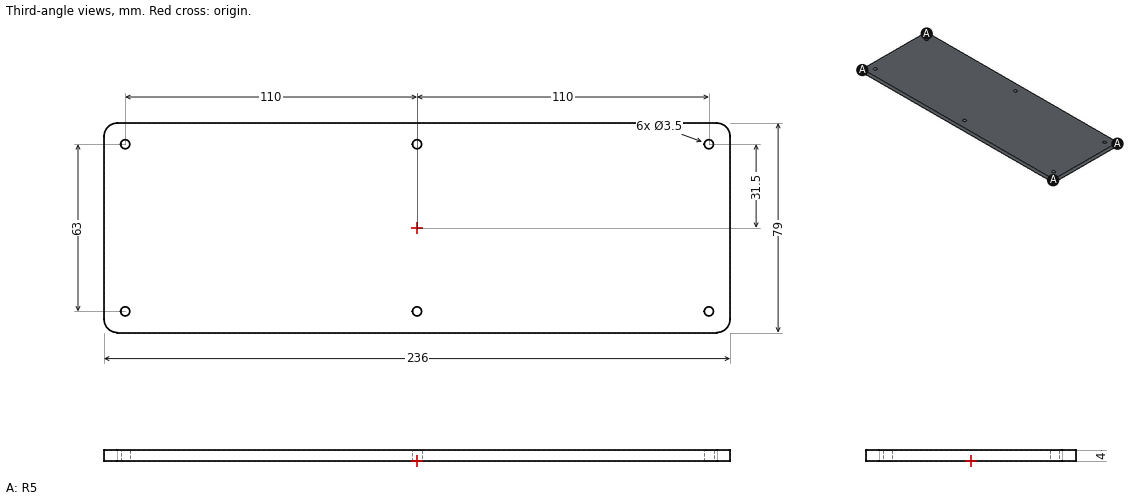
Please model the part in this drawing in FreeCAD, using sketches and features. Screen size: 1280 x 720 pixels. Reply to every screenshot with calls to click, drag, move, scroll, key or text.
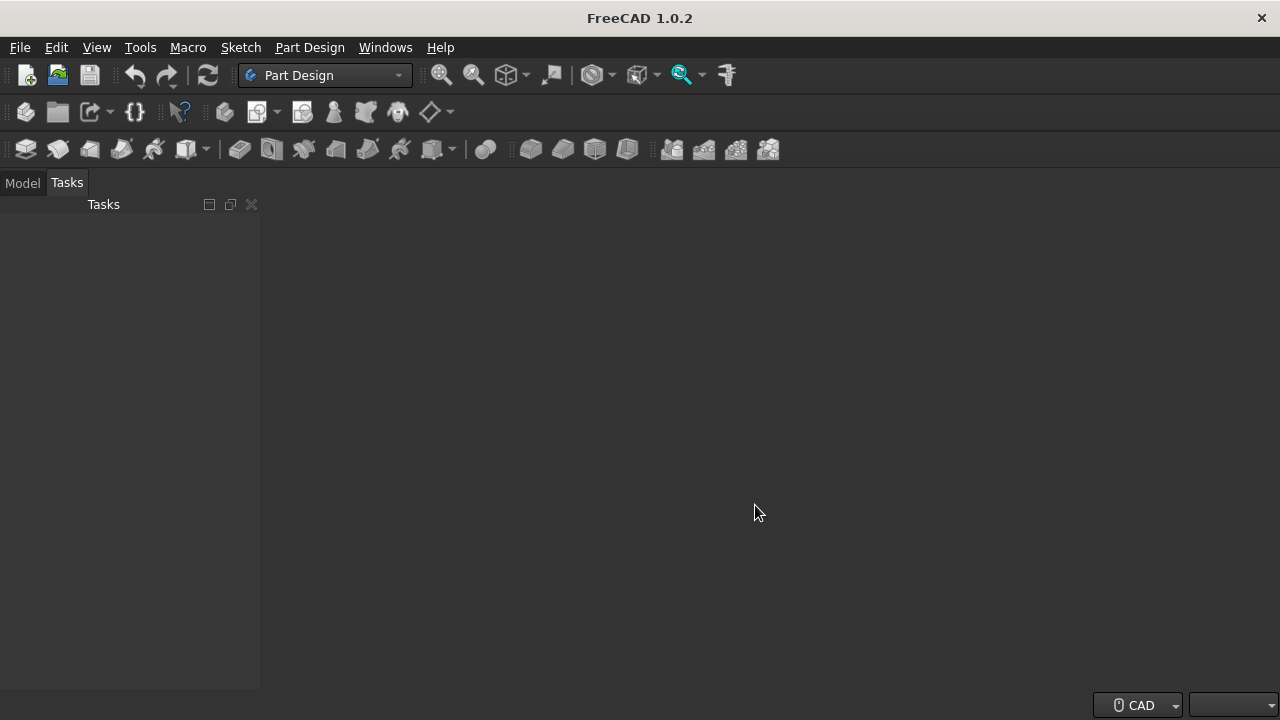
click(26, 76)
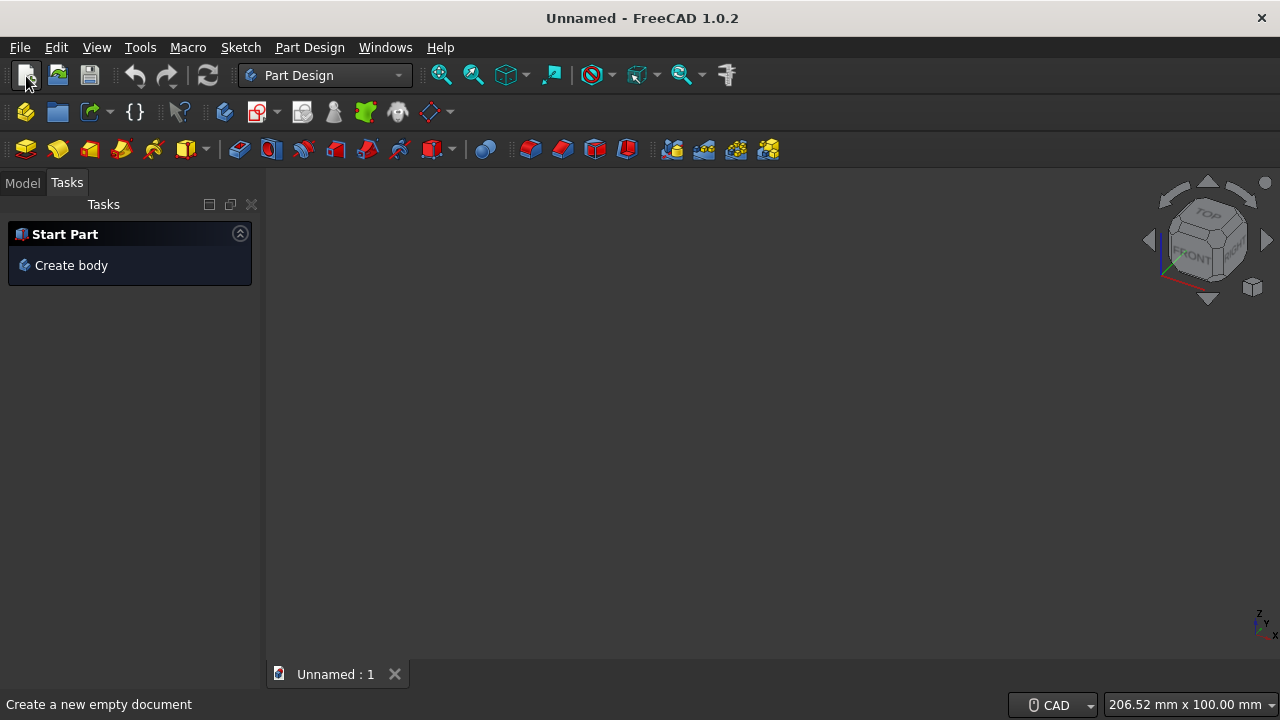
click(258, 112)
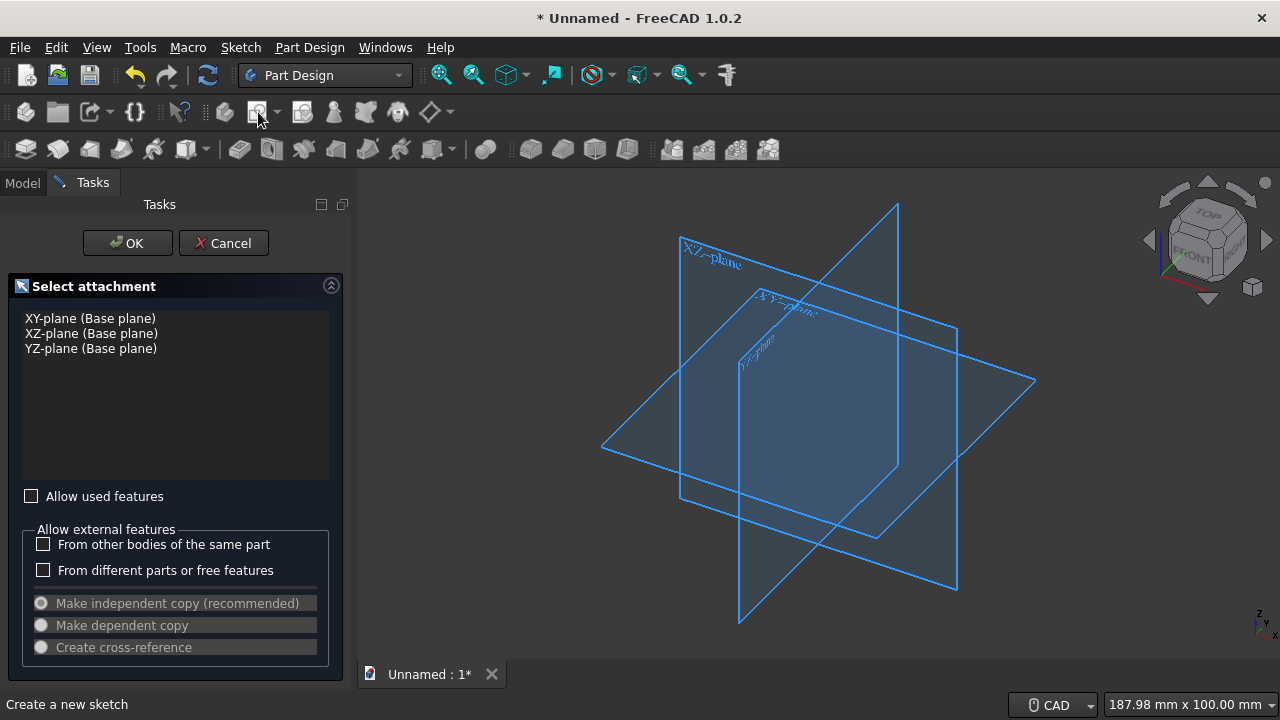
click(82, 318)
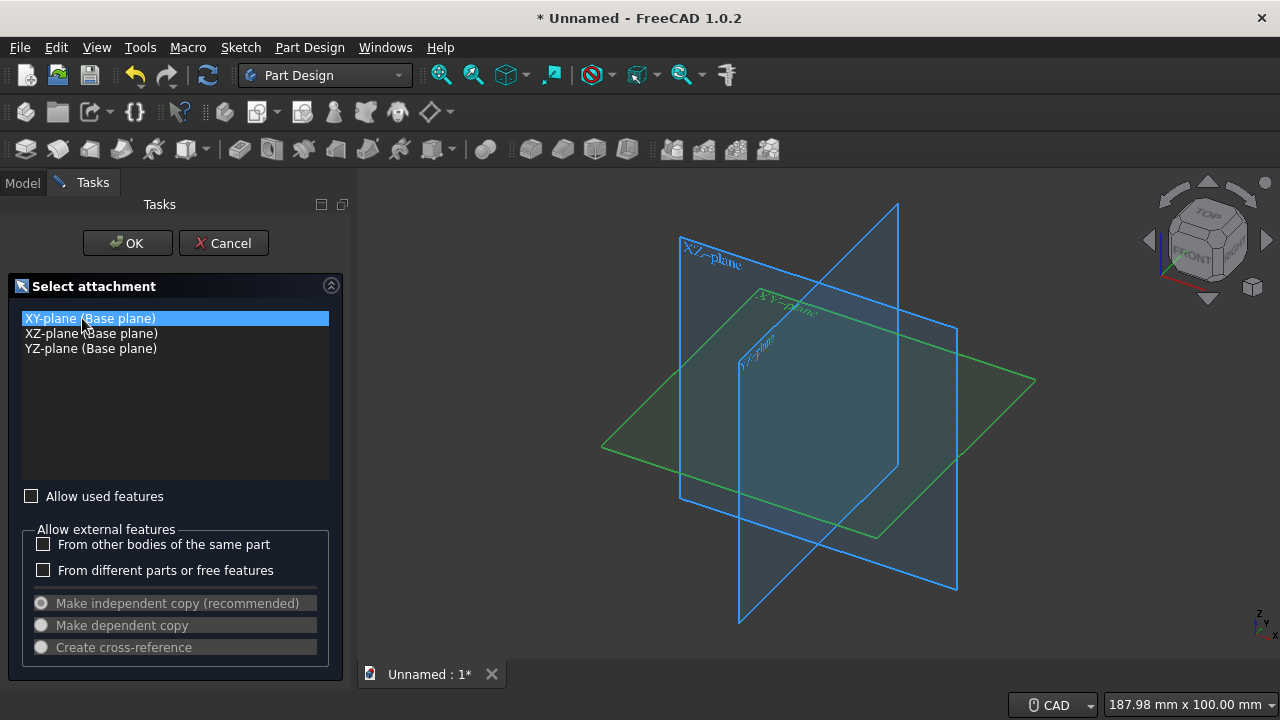
click(128, 243)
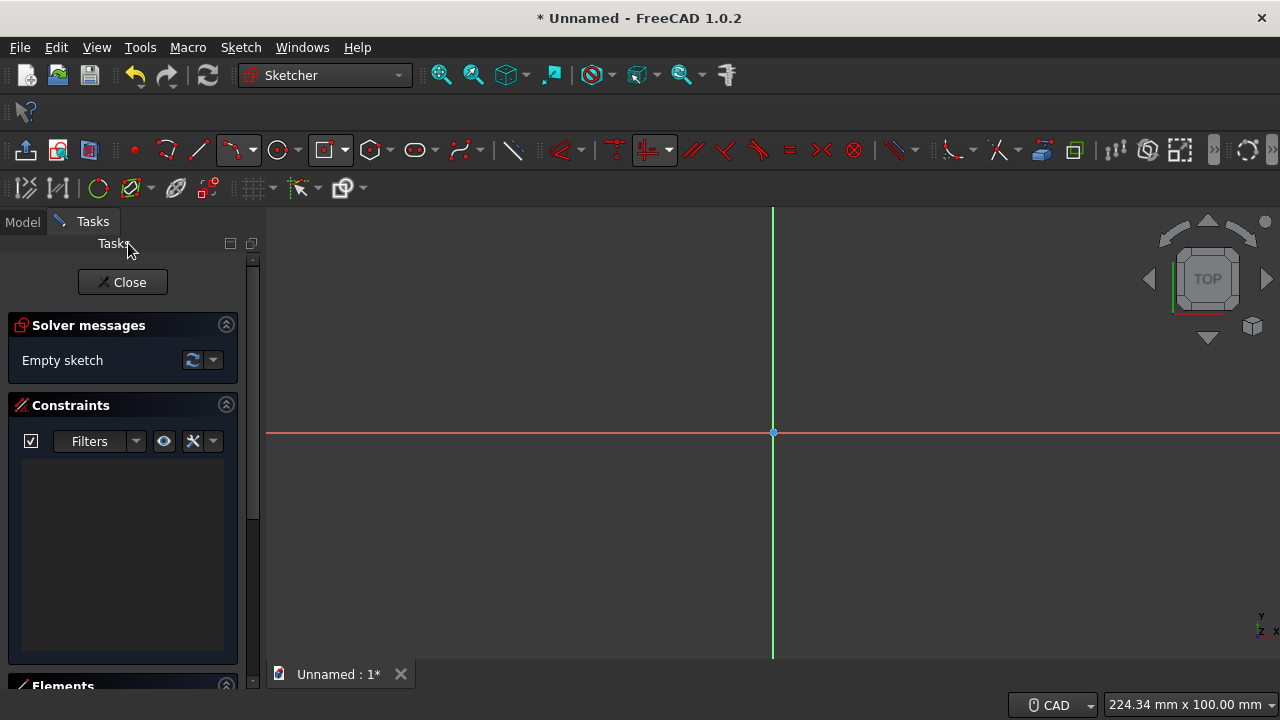
scroll(621, 433, down, 3)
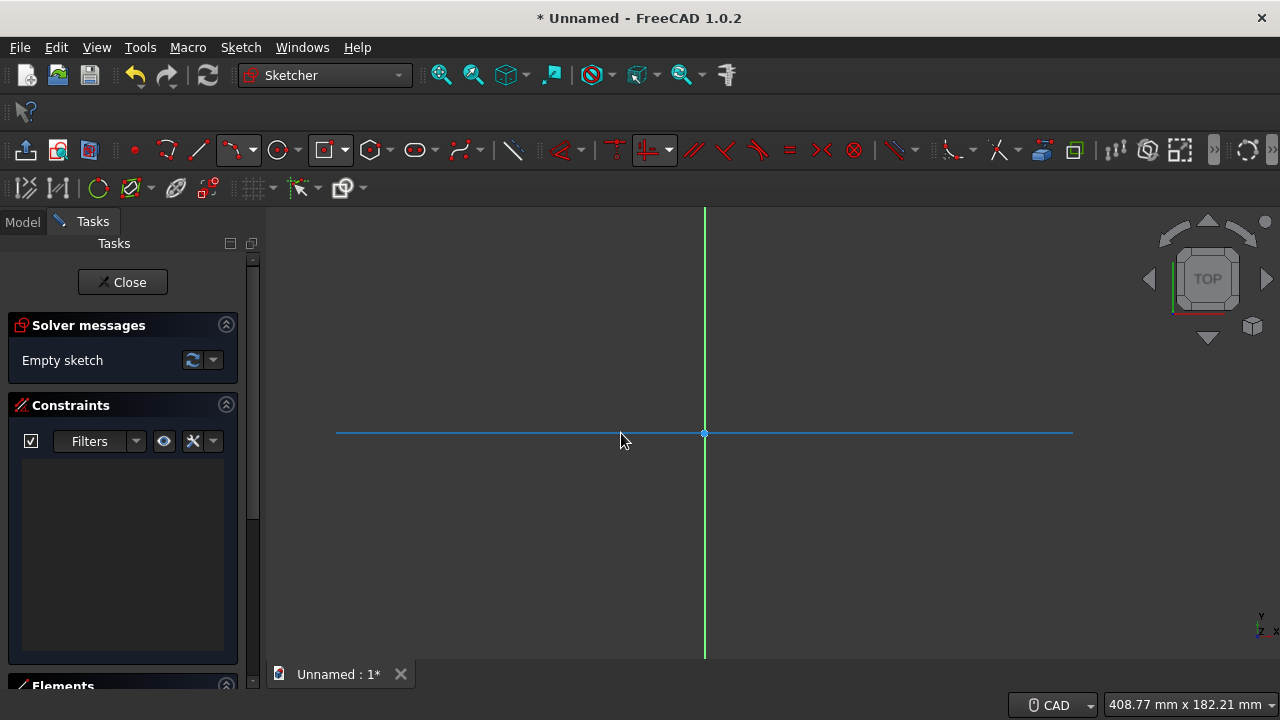
click(324, 150)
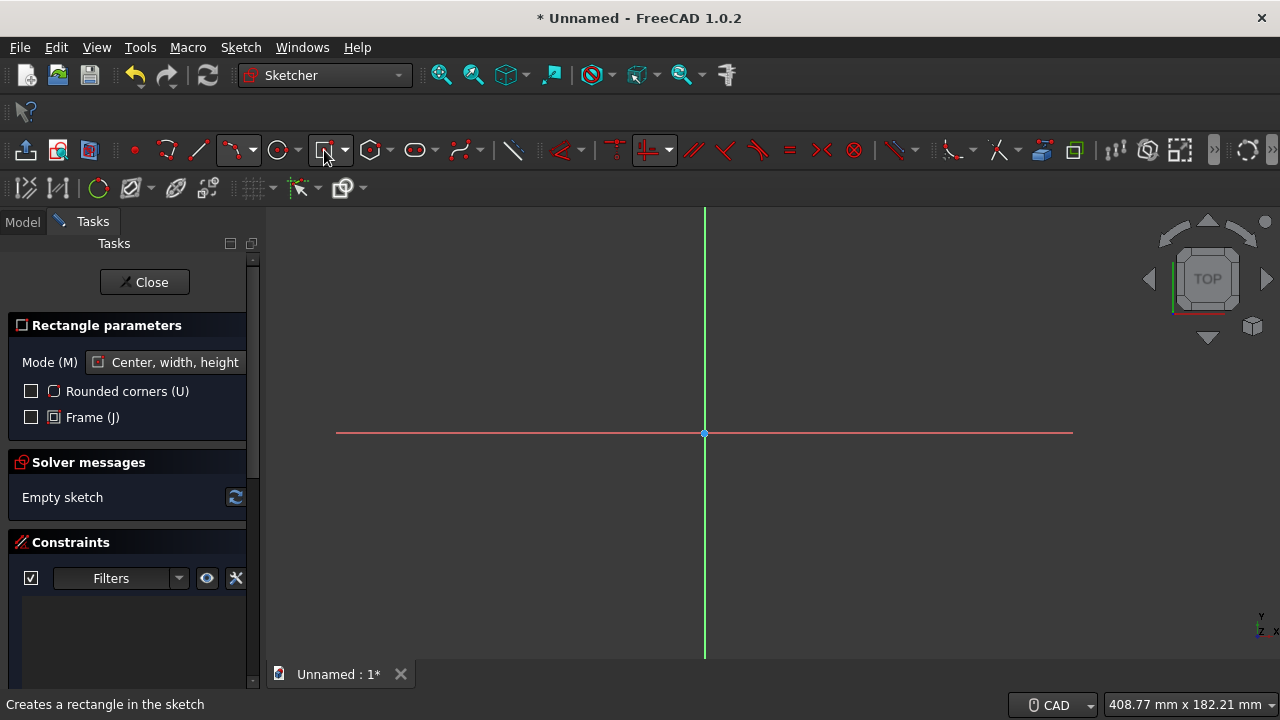
click(705, 433)
move(997, 335)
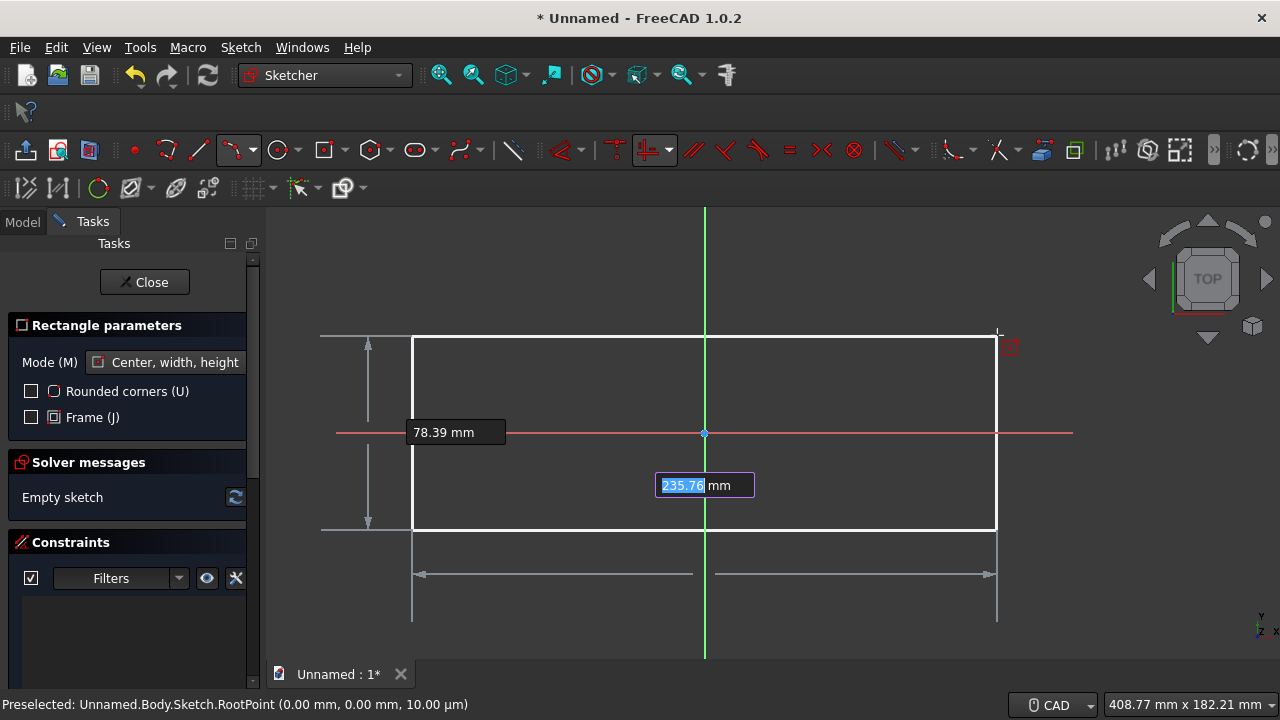
text(236)
key(Tab)
text(79)
key(Return)
key(Escape)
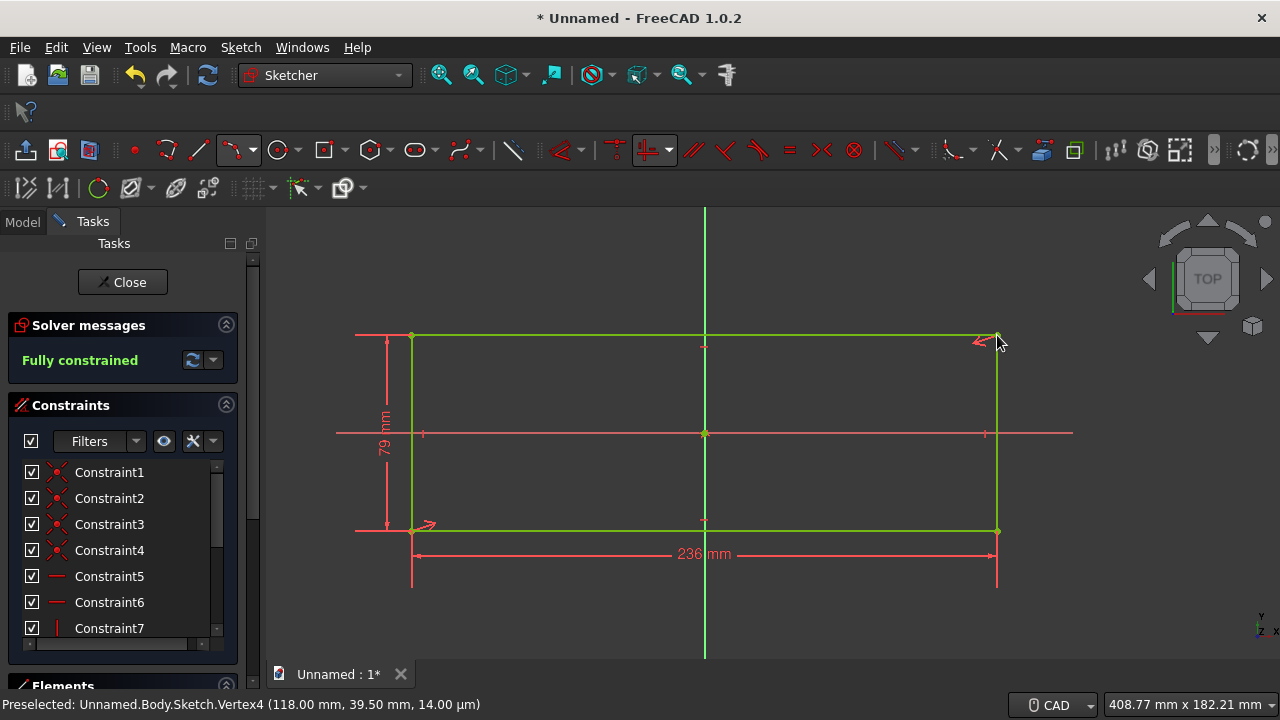
click(123, 282)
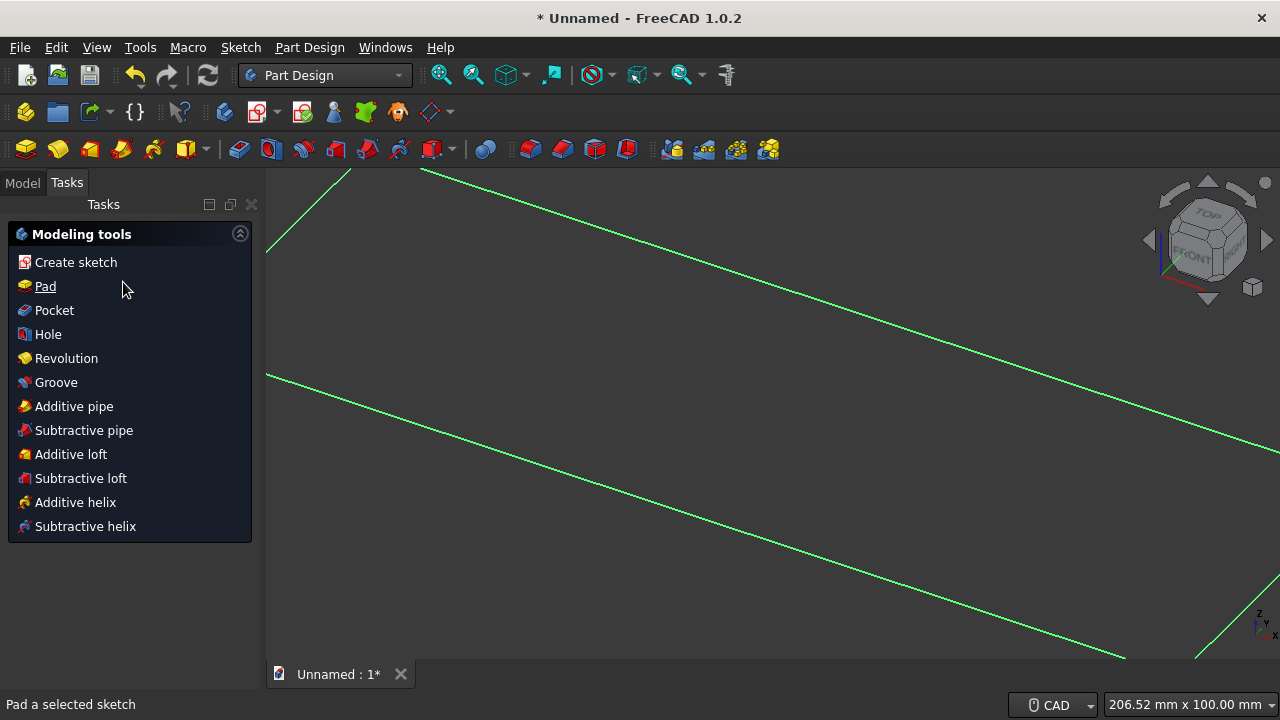
click(26, 150)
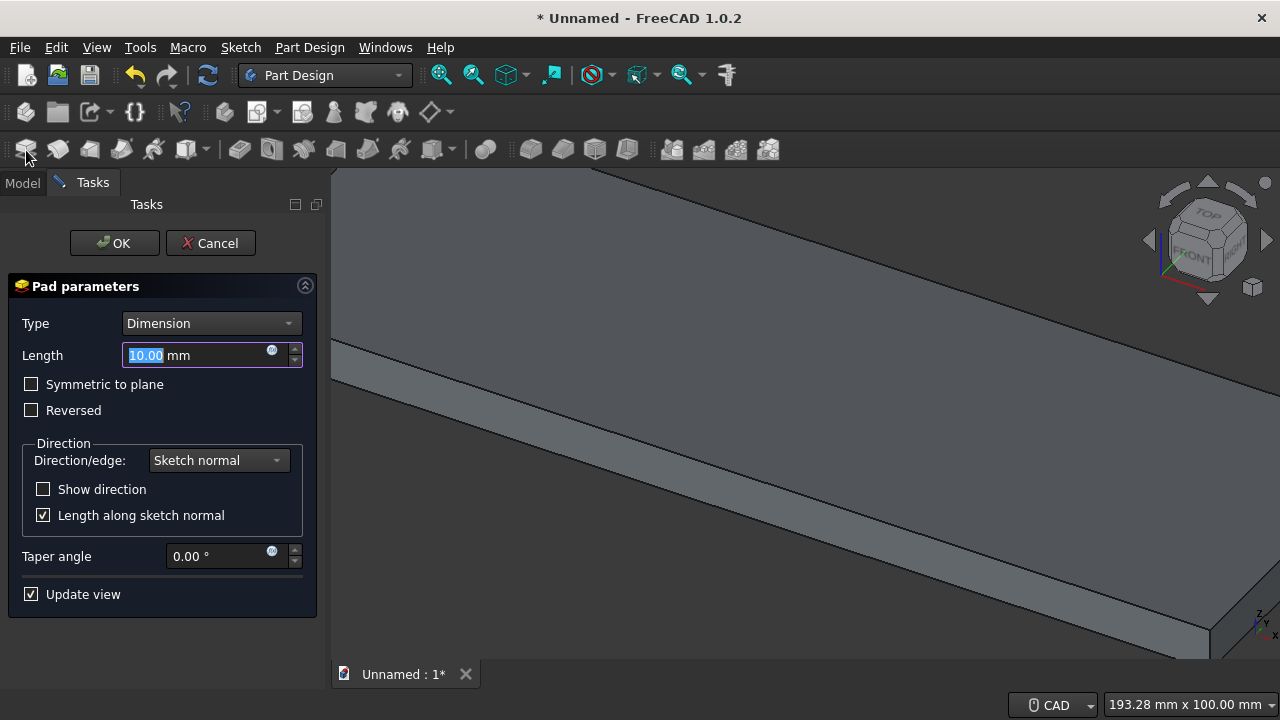
text(4)
key(Tab)